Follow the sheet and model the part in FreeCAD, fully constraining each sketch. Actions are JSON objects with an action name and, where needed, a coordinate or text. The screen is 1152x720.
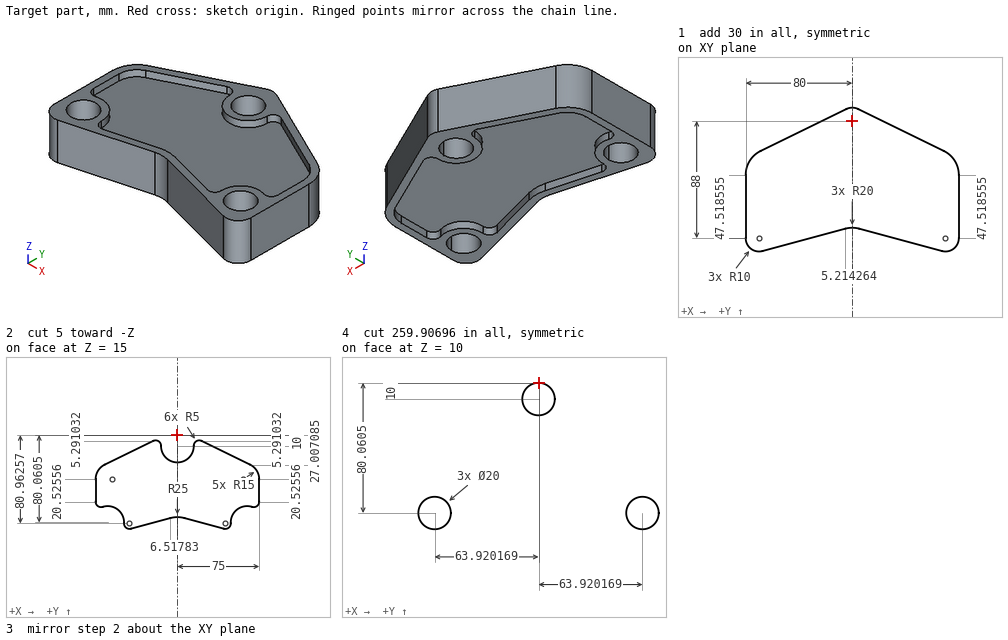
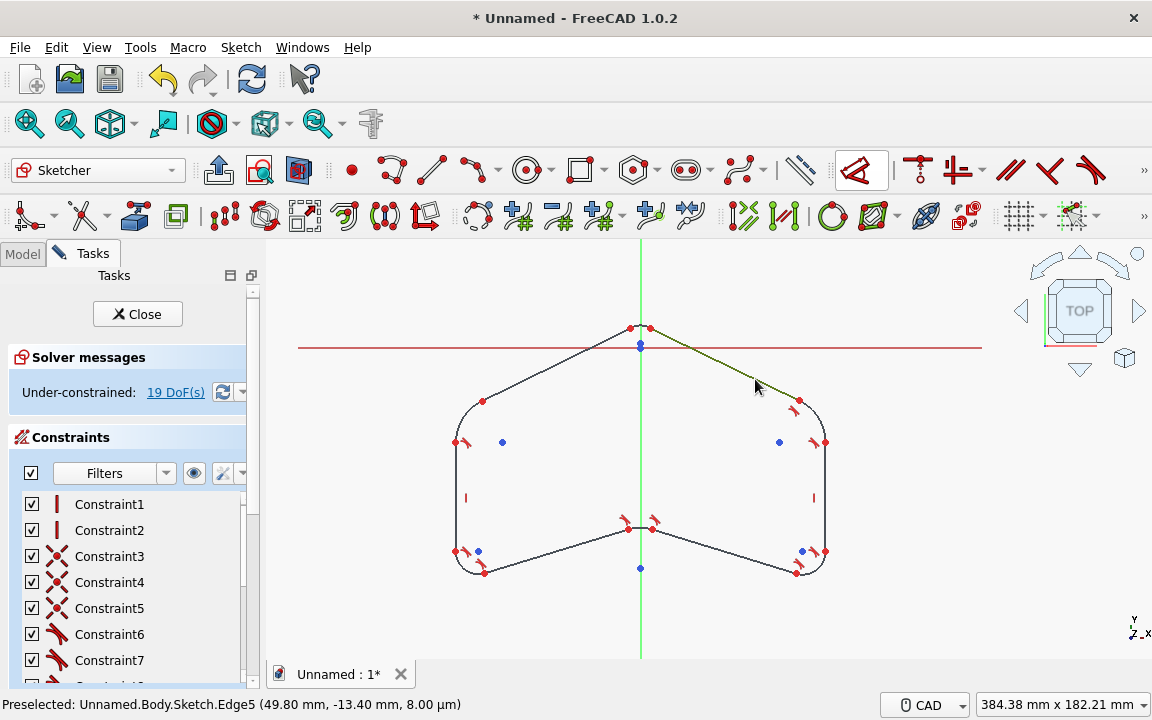
{"action": "scroll", "coordinate": [640, 325], "scroll_direction": "up", "scroll_amount": 2}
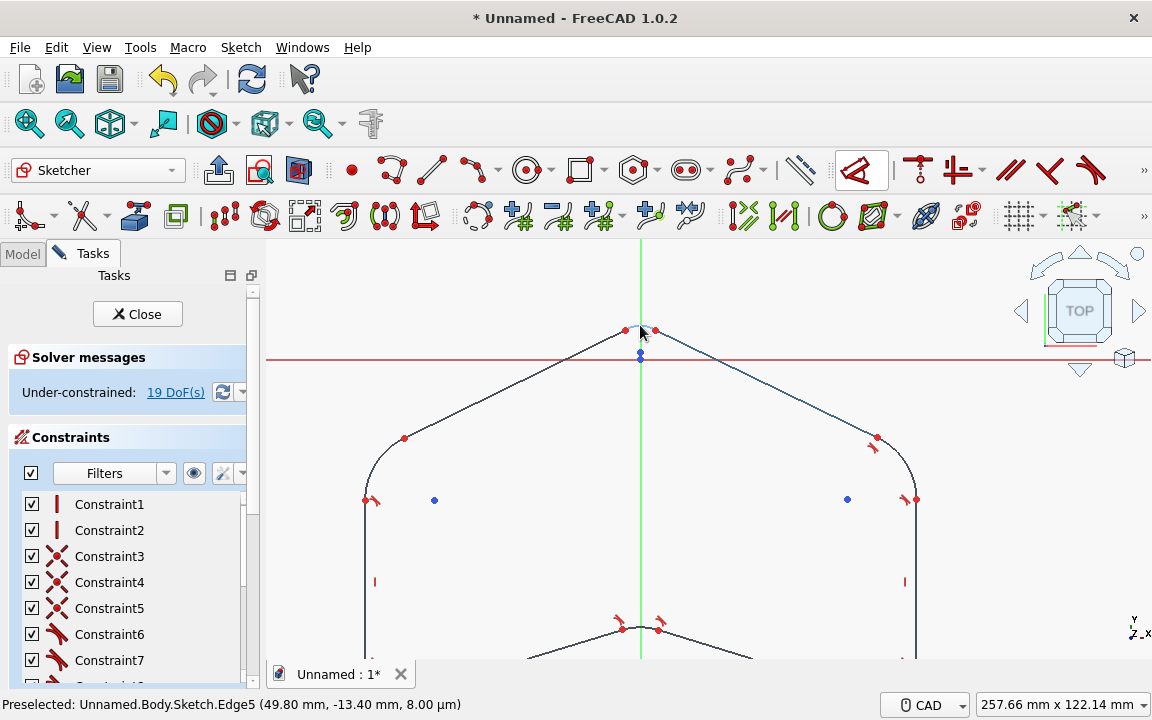
{"action": "left_click", "coordinate": [640, 326]}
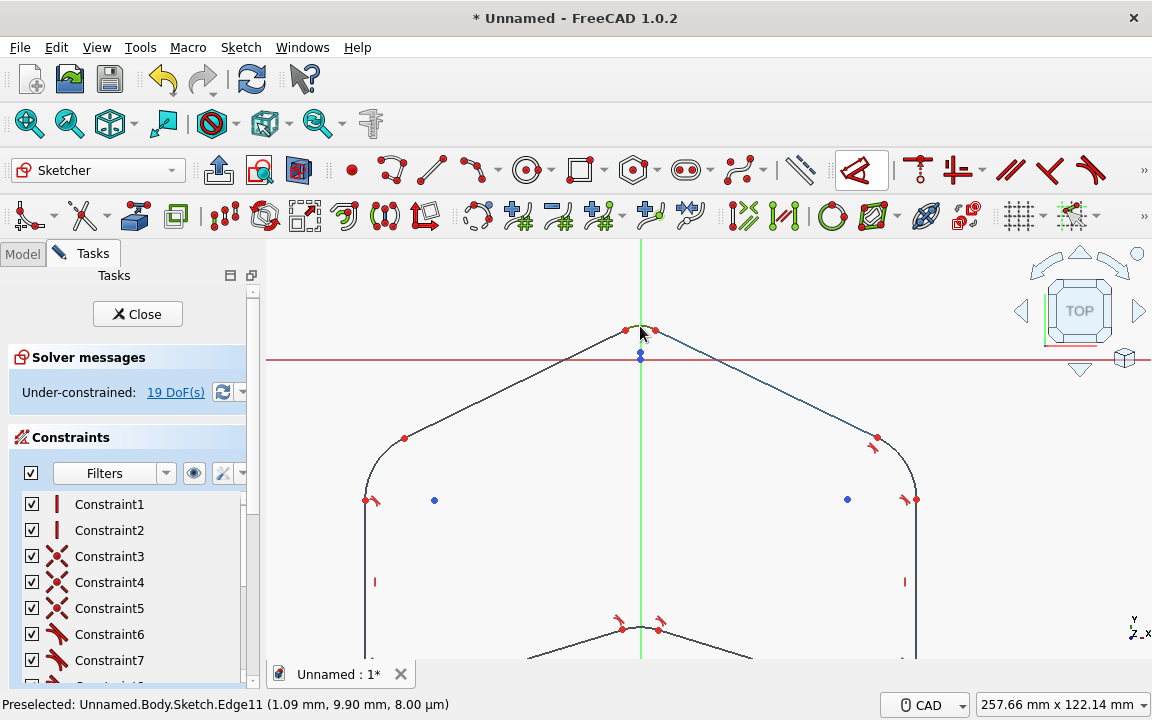
{"action": "key", "text": "t"}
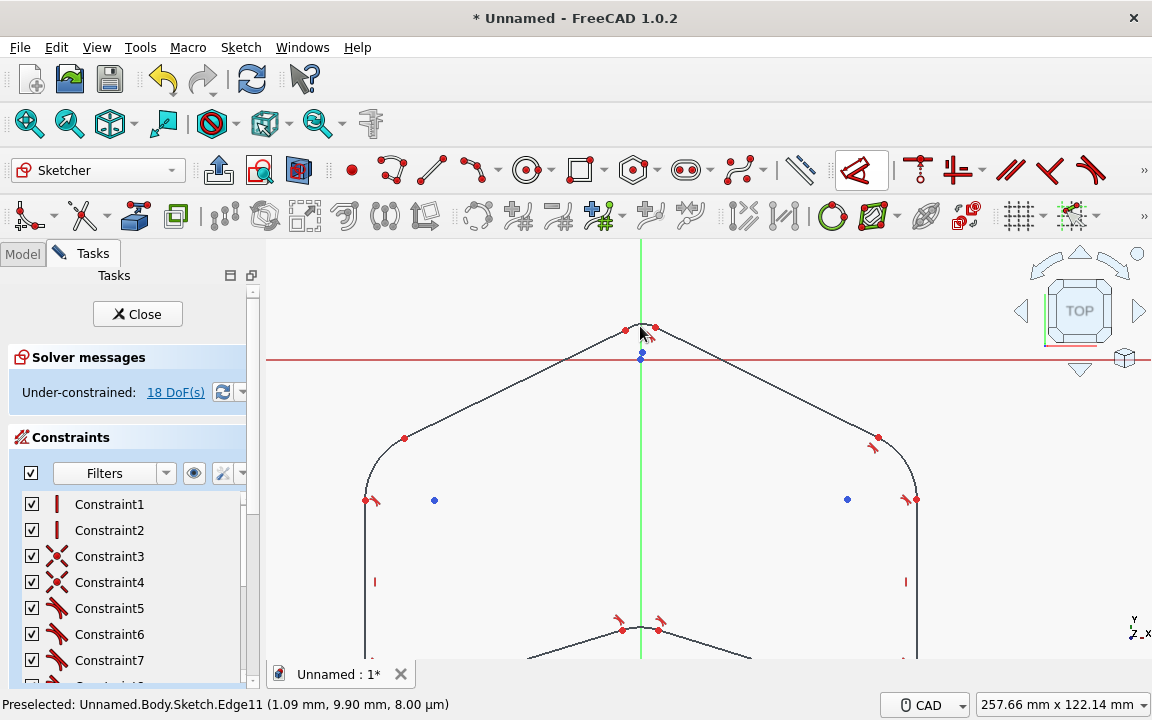
{"action": "left_click", "coordinate": [559, 363]}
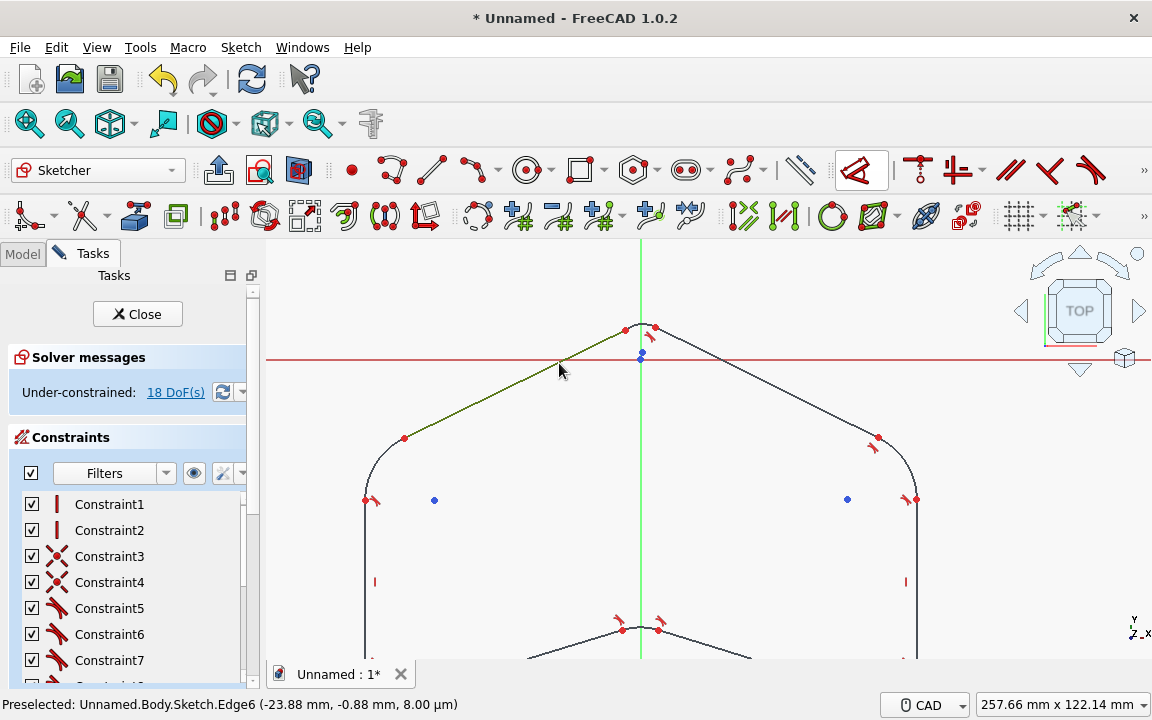
{"action": "left_click", "coordinate": [640, 324]}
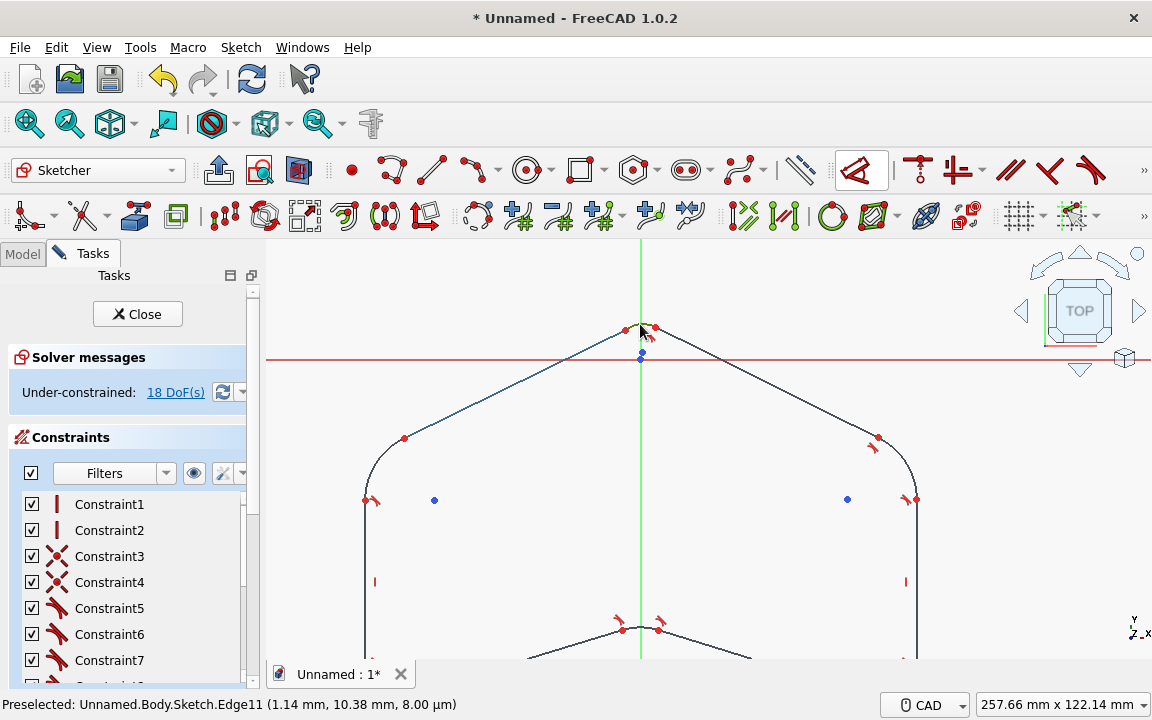
{"action": "key", "text": "t"}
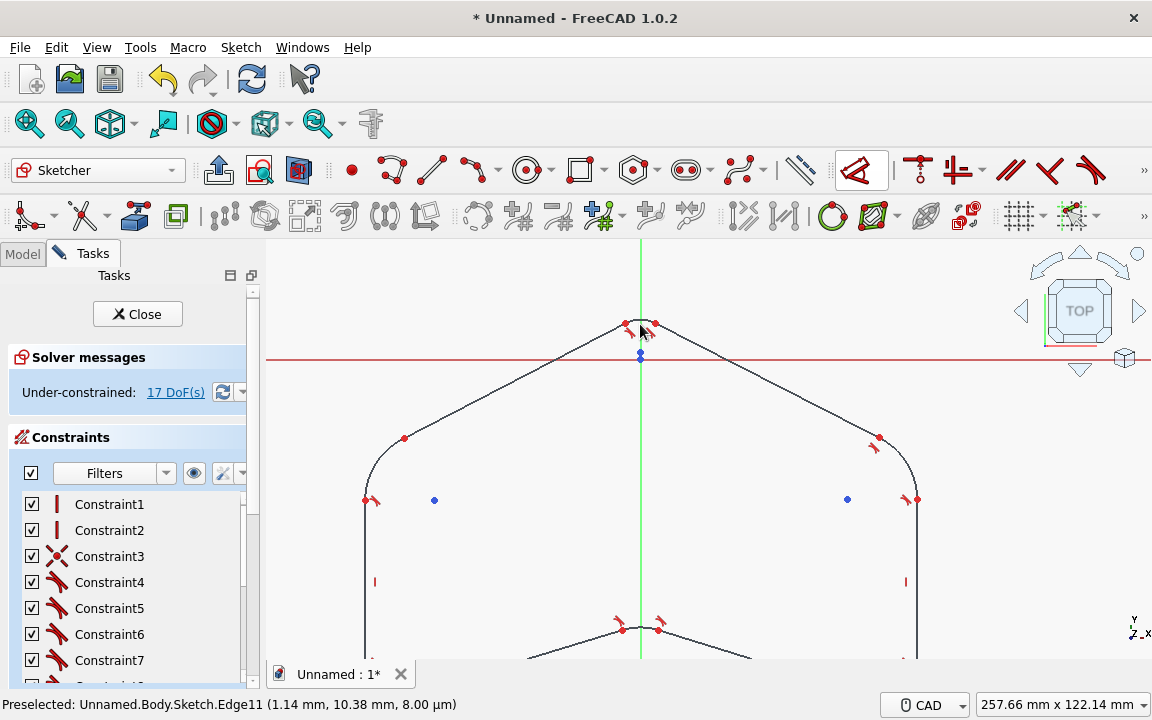
{"action": "left_click", "coordinate": [559, 358]}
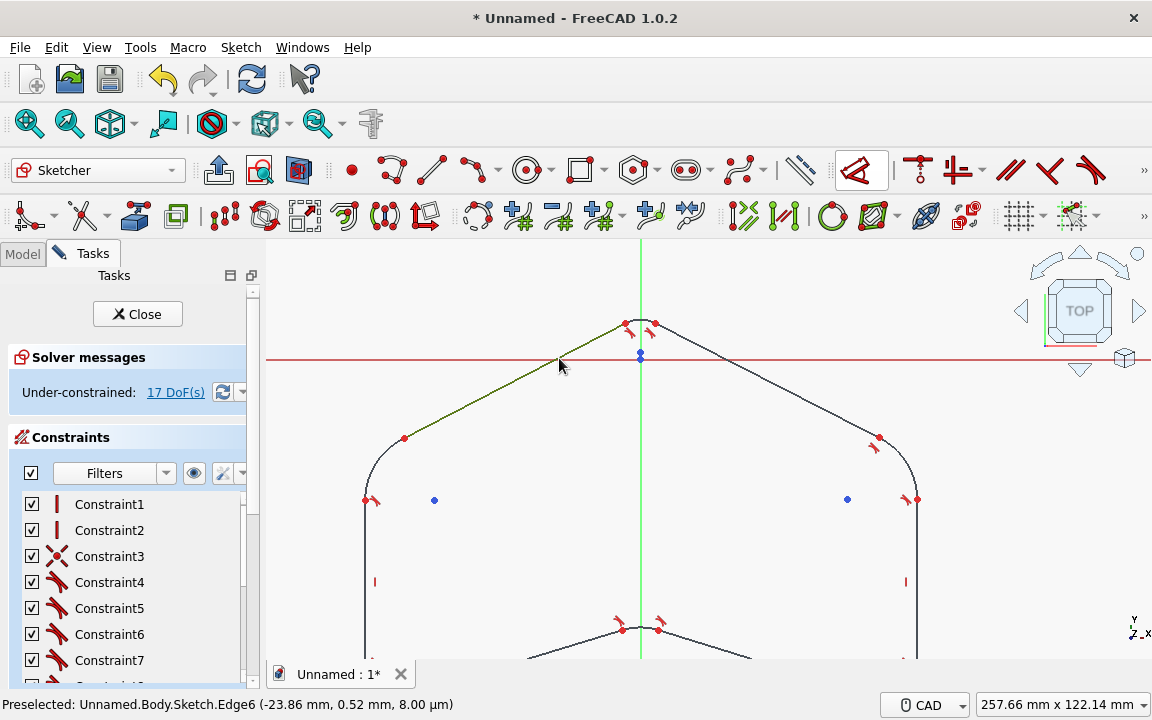
{"action": "left_click", "coordinate": [385, 452]}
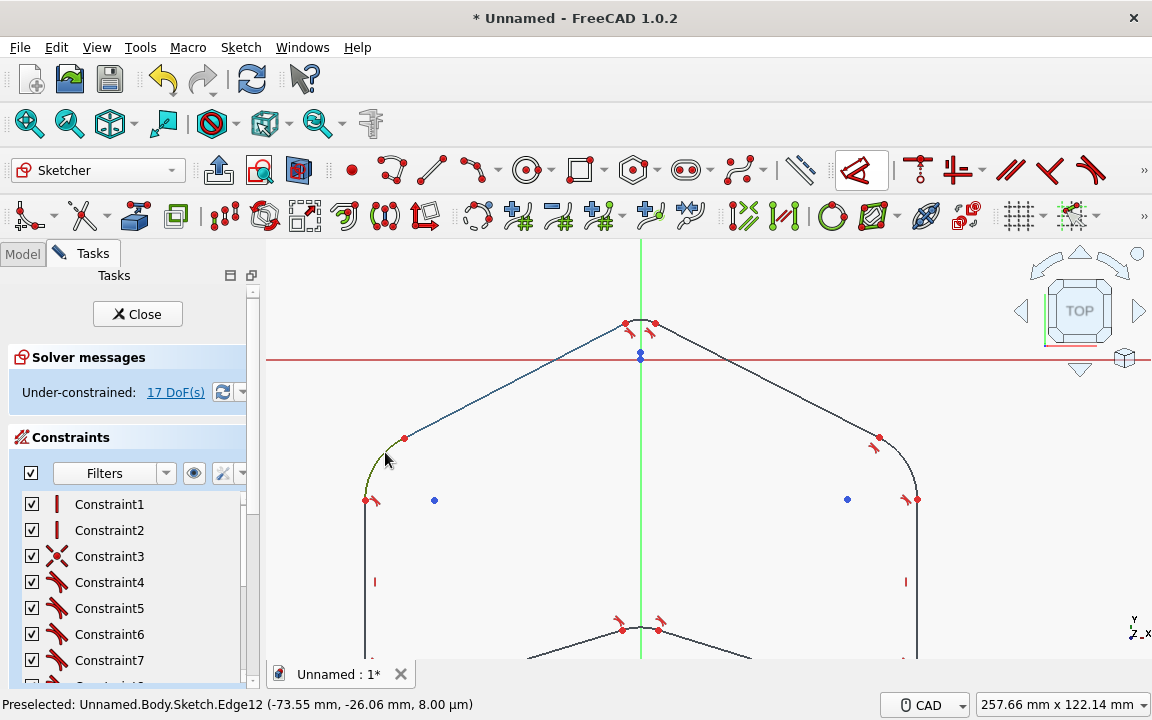
{"action": "left_click", "coordinate": [1092, 170]}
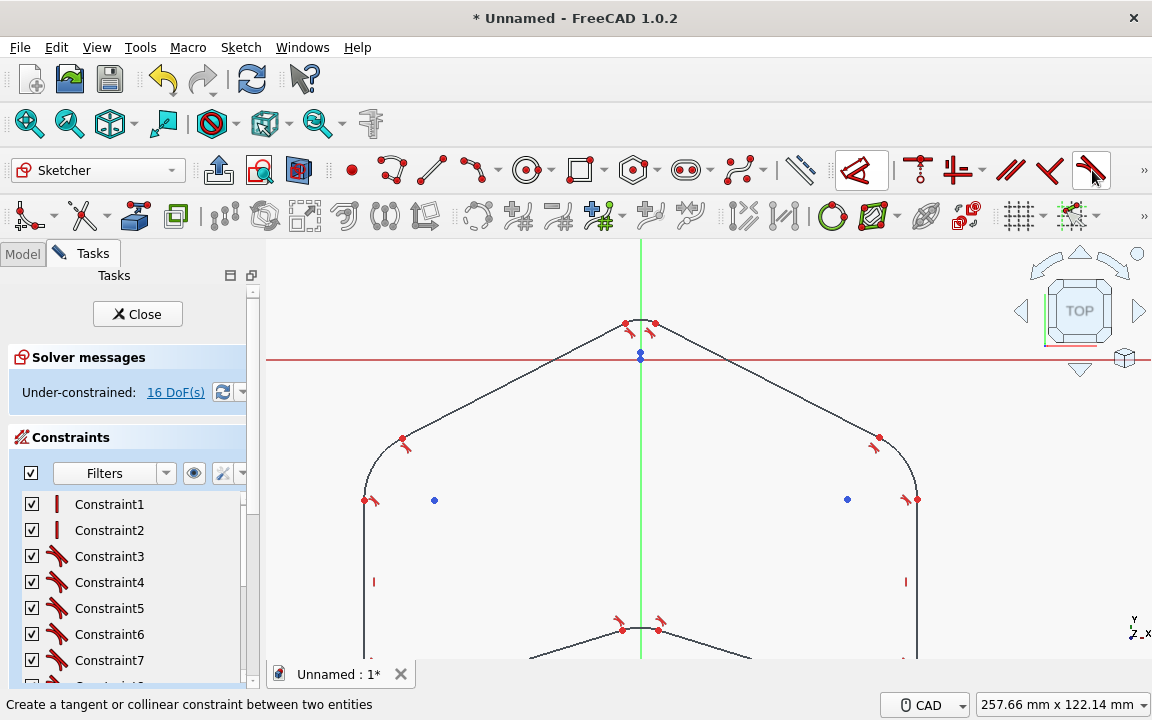
{"action": "left_click_drag", "start_coordinate": [631, 343], "coordinate": [651, 370]}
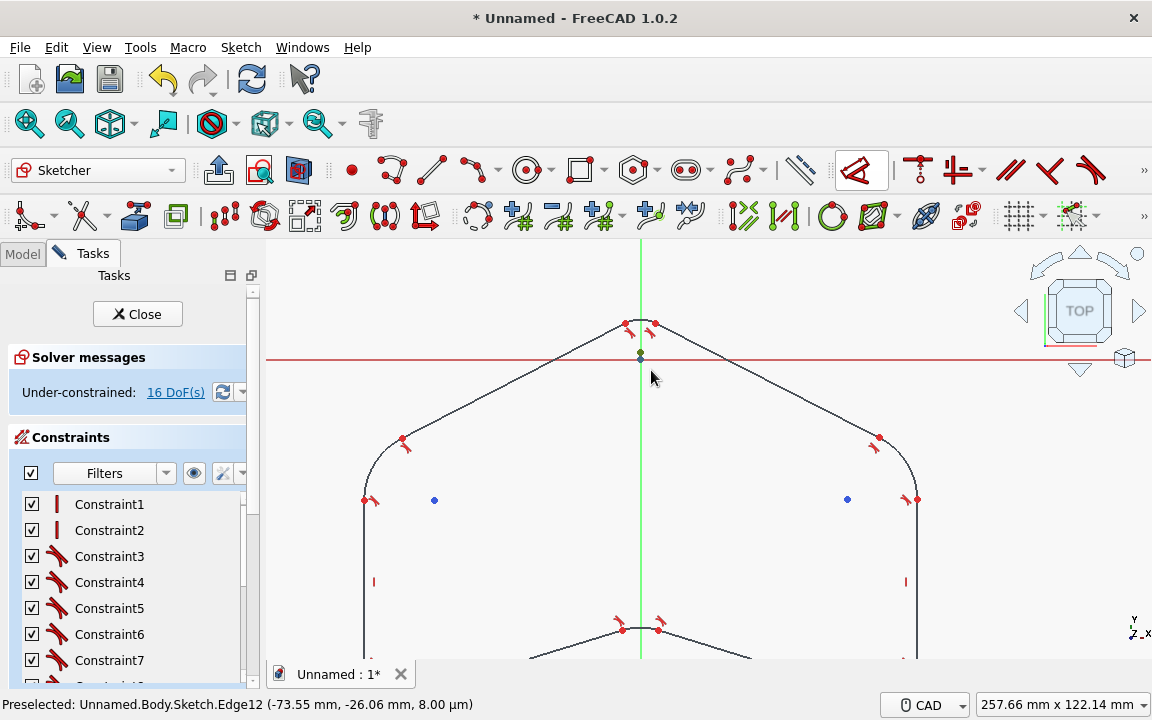
{"action": "left_click", "coordinate": [918, 170]}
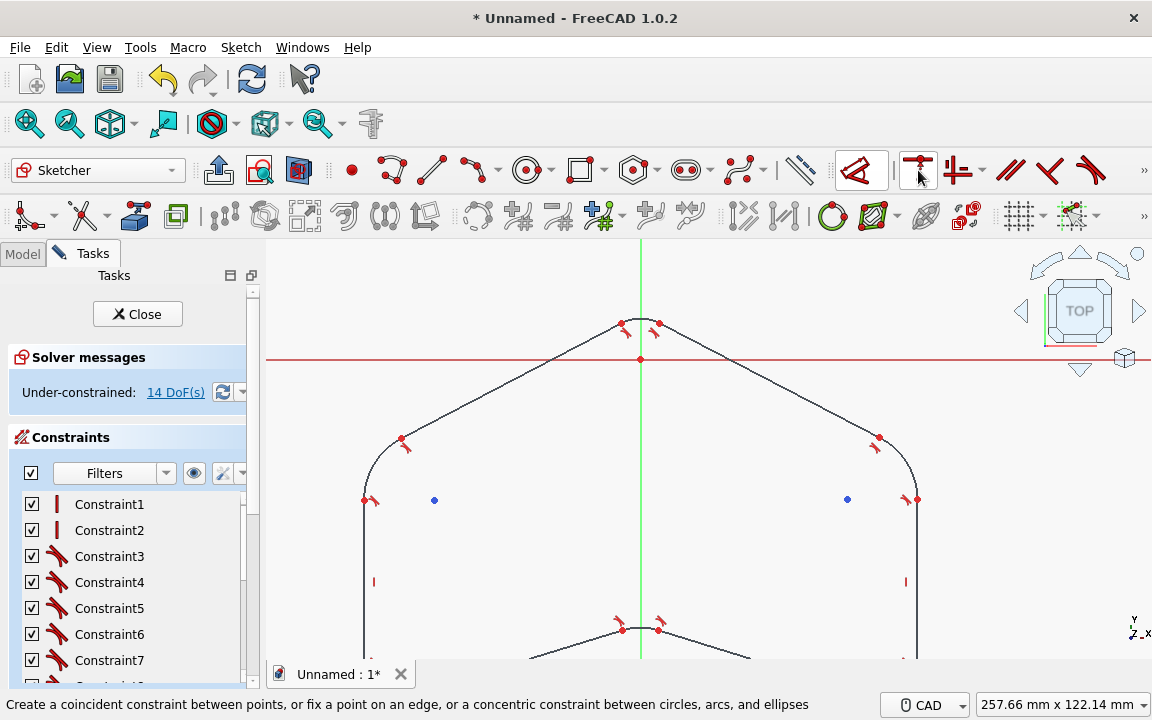
{"action": "scroll", "coordinate": [640, 324], "scroll_direction": "down", "scroll_amount": 2}